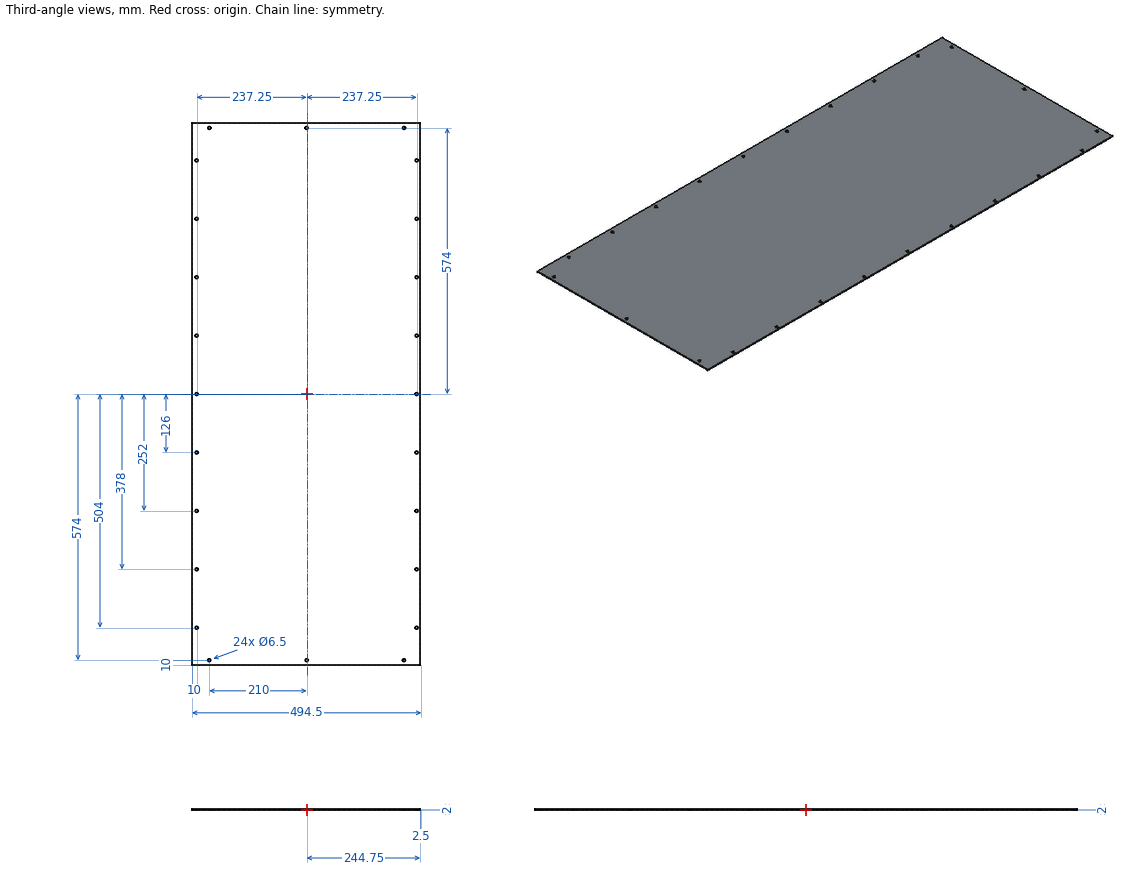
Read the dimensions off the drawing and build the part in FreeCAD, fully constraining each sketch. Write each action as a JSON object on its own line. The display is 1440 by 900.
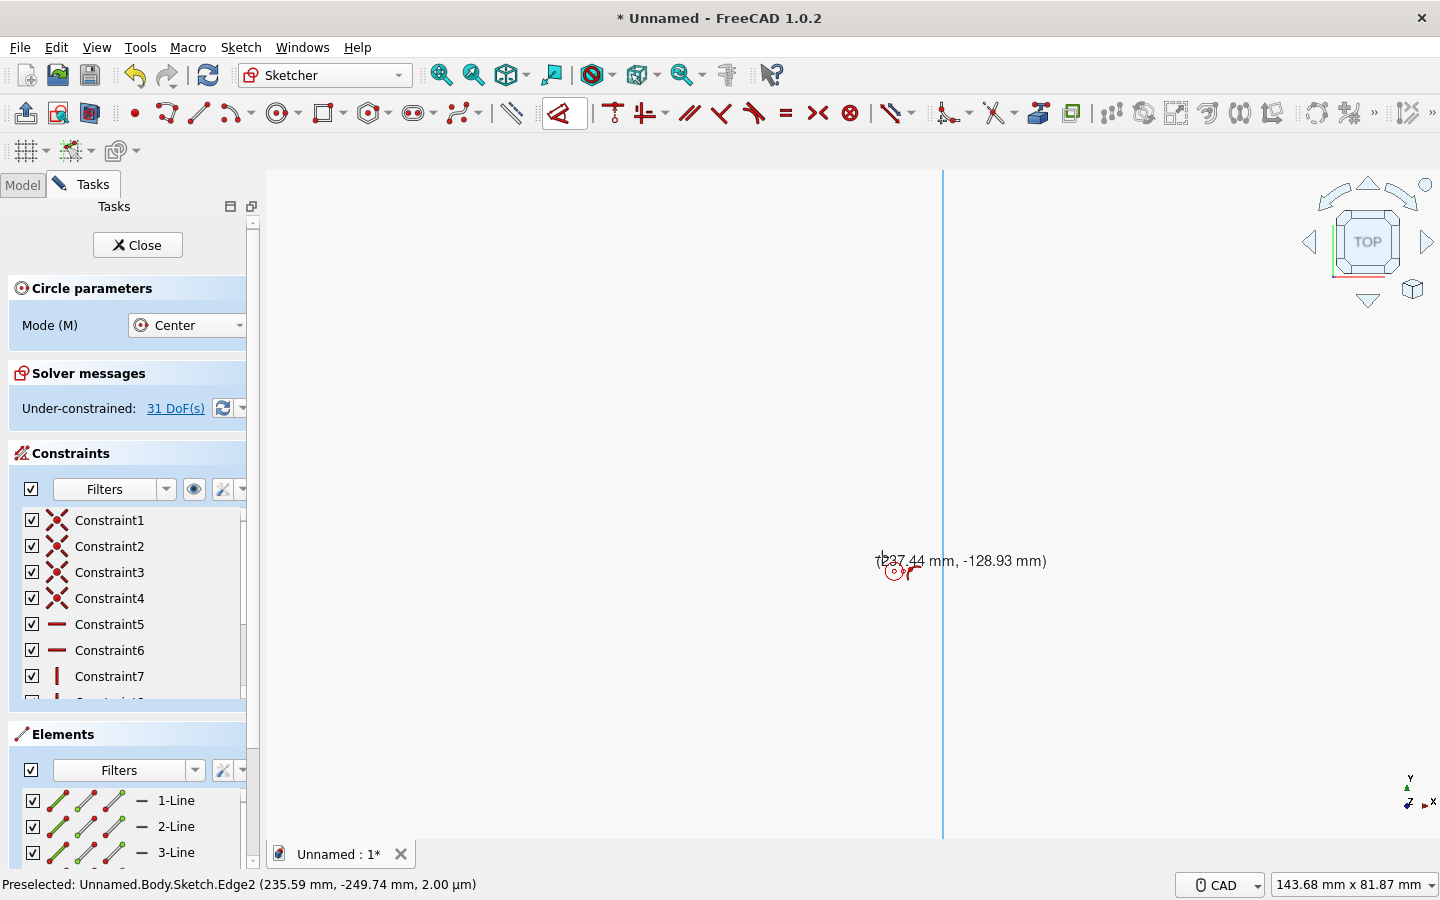
{"action": "scroll", "coordinate": [882, 556], "scroll_direction": "down", "scroll_amount": 15}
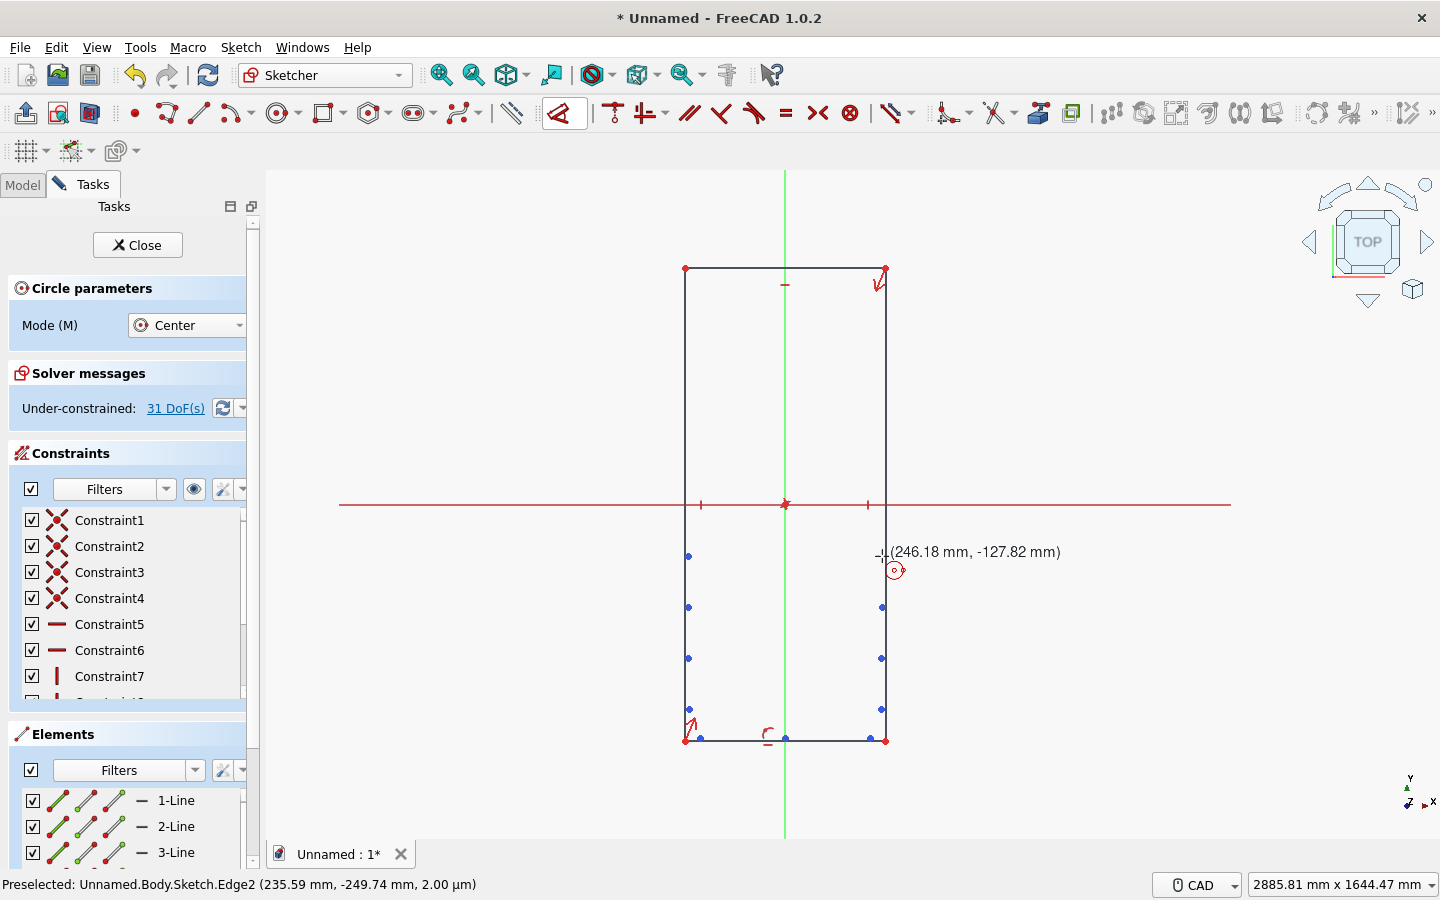
{"action": "scroll", "coordinate": [882, 556], "scroll_direction": "up", "scroll_amount": 7}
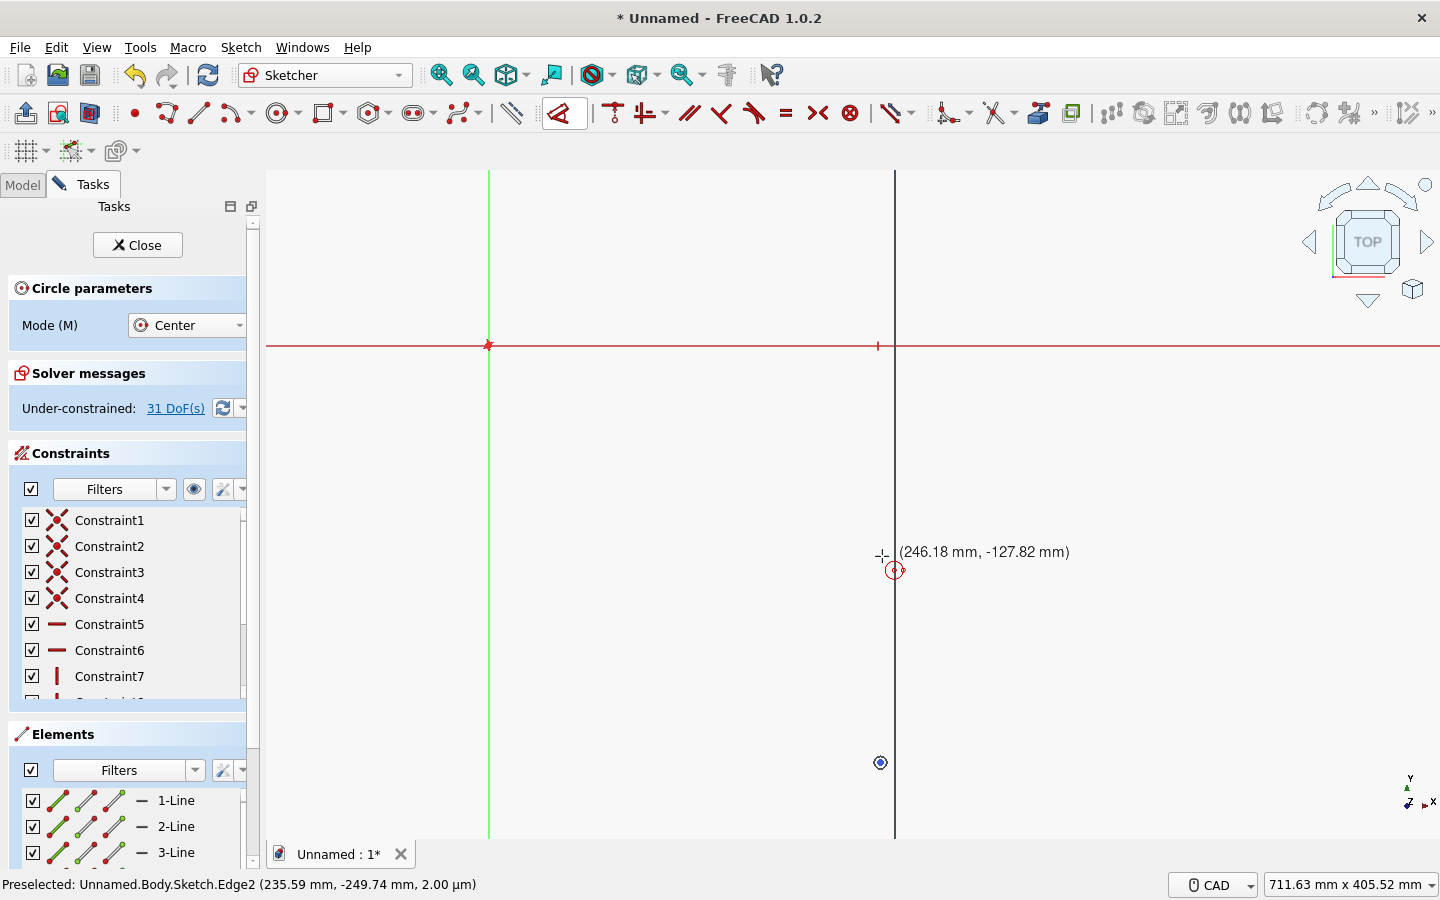
{"action": "left_click", "coordinate": [880, 554]}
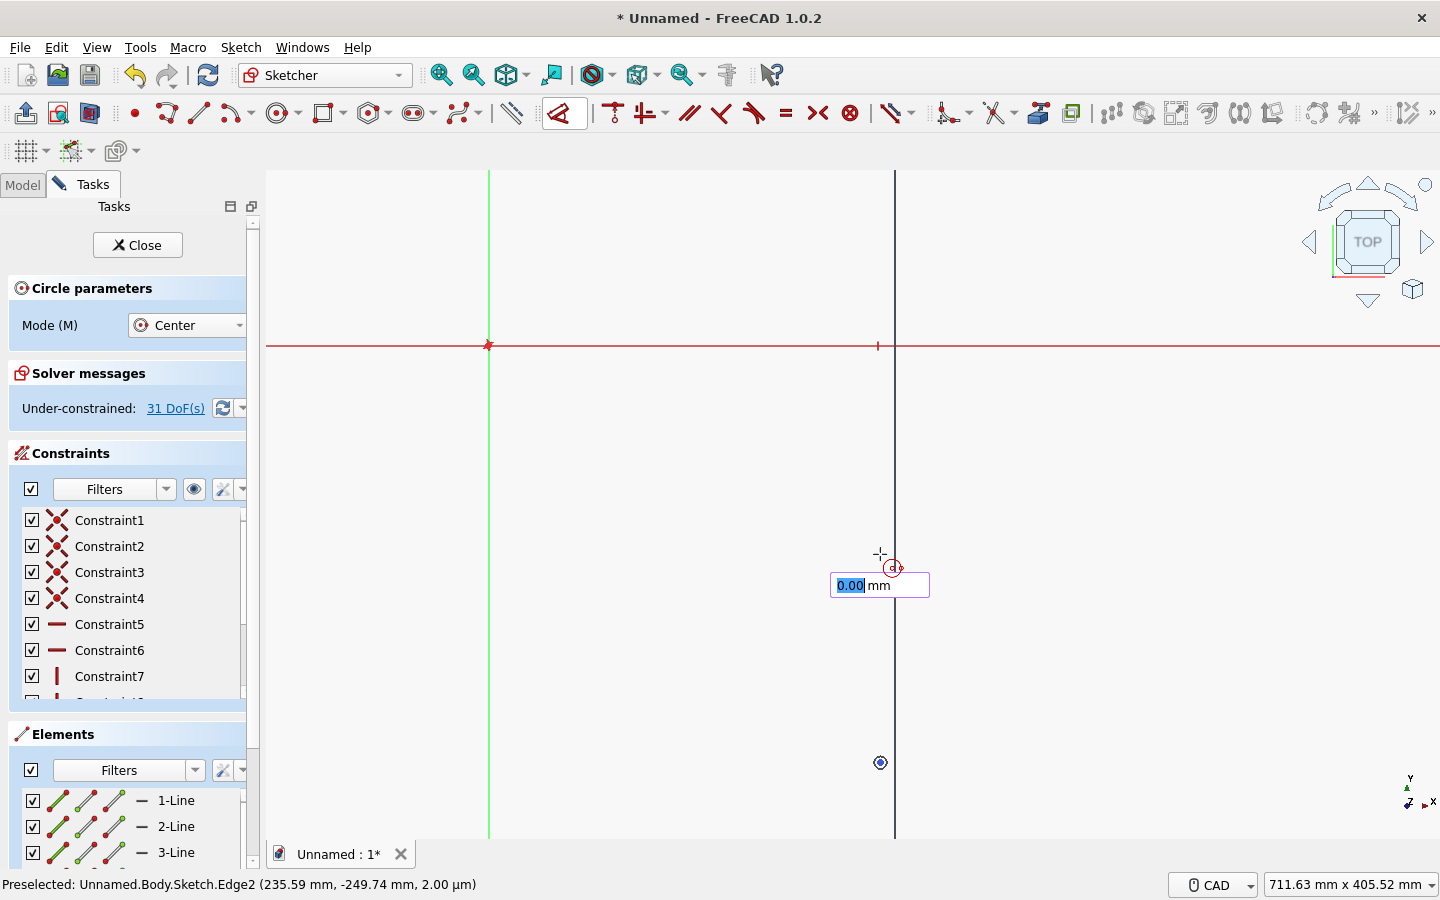
{"action": "scroll", "coordinate": [876, 550], "scroll_direction": "up", "scroll_amount": 6}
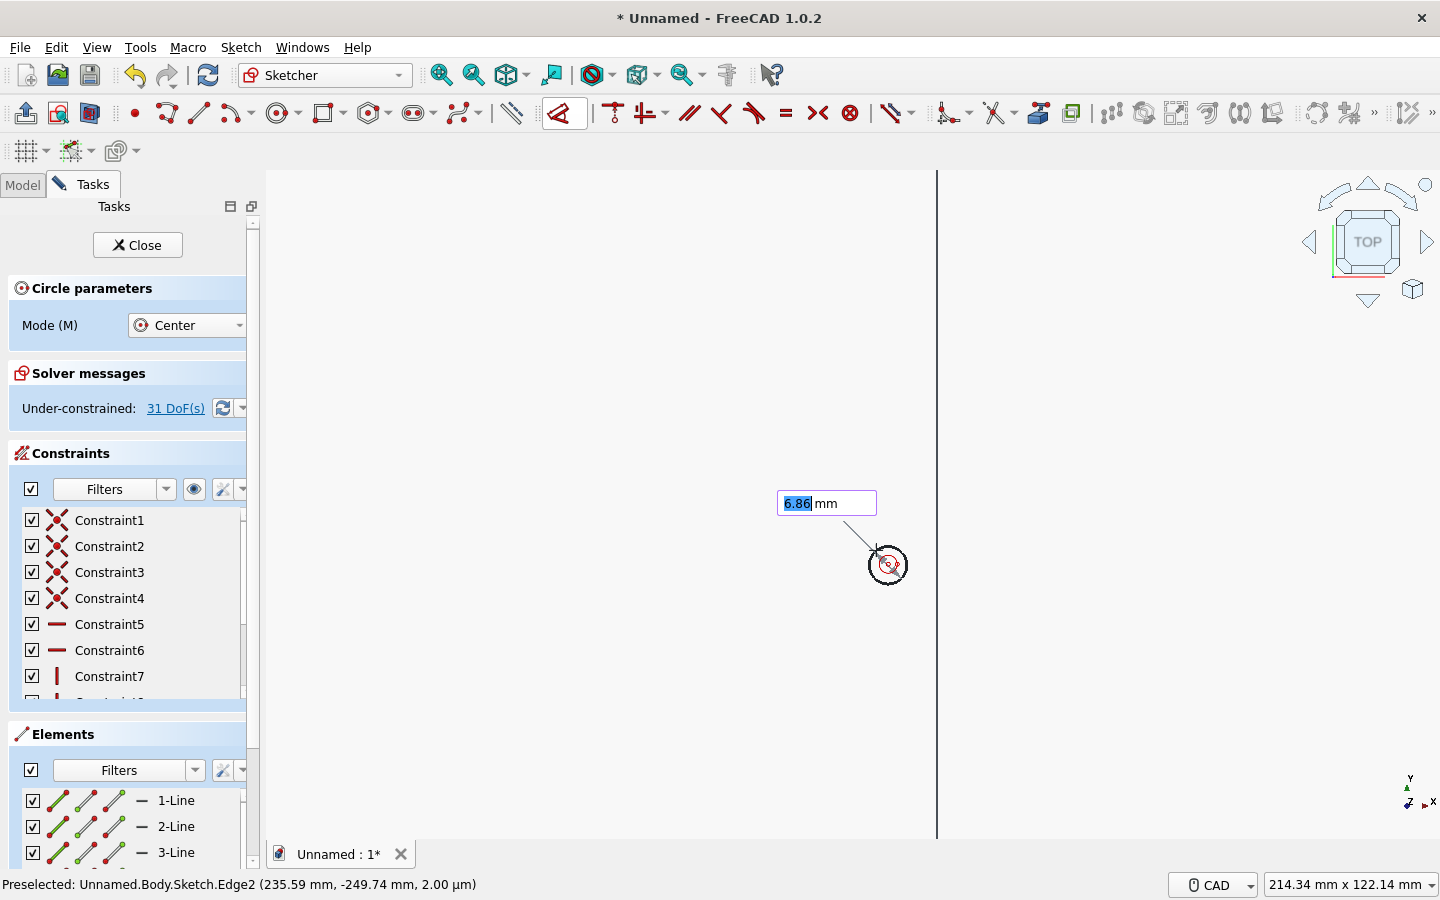
{"action": "left_click", "coordinate": [876, 548]}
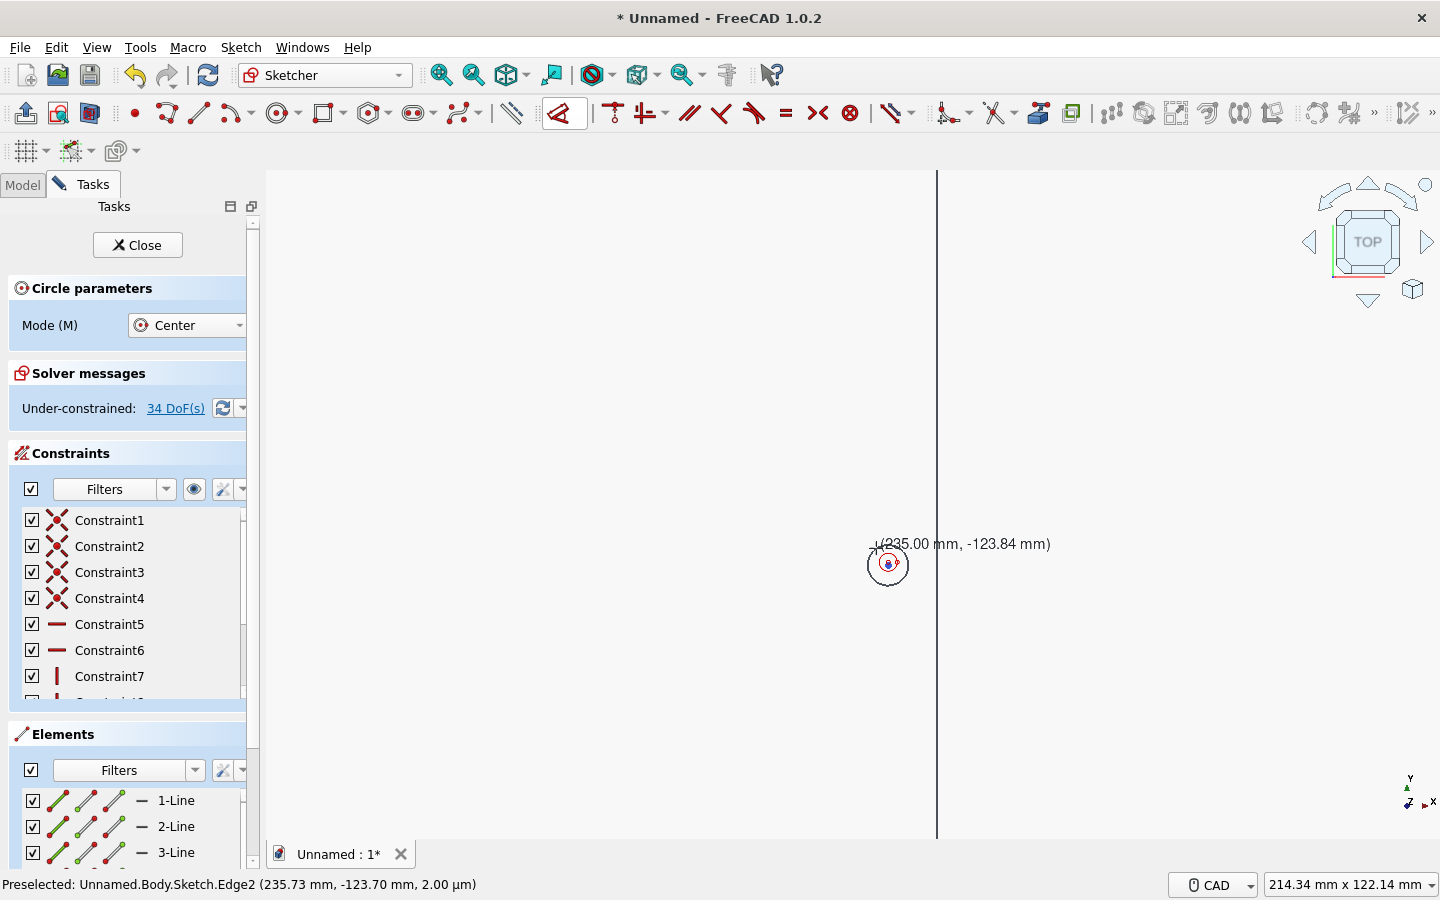
{"action": "scroll", "coordinate": [880, 555], "scroll_direction": "down", "scroll_amount": 13}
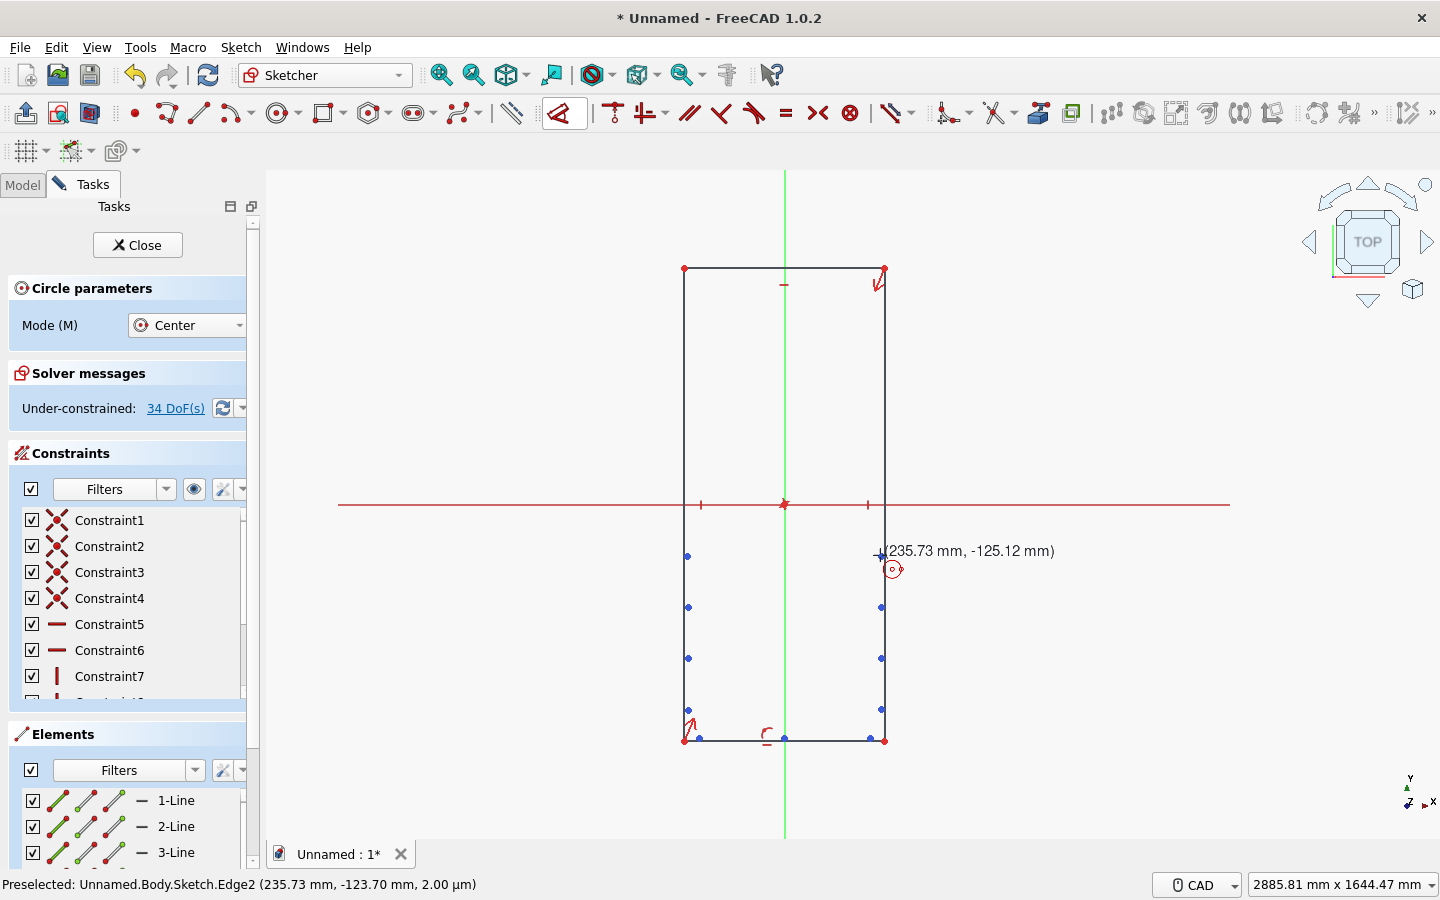
{"action": "scroll", "coordinate": [688, 505], "scroll_direction": "up", "scroll_amount": 15}